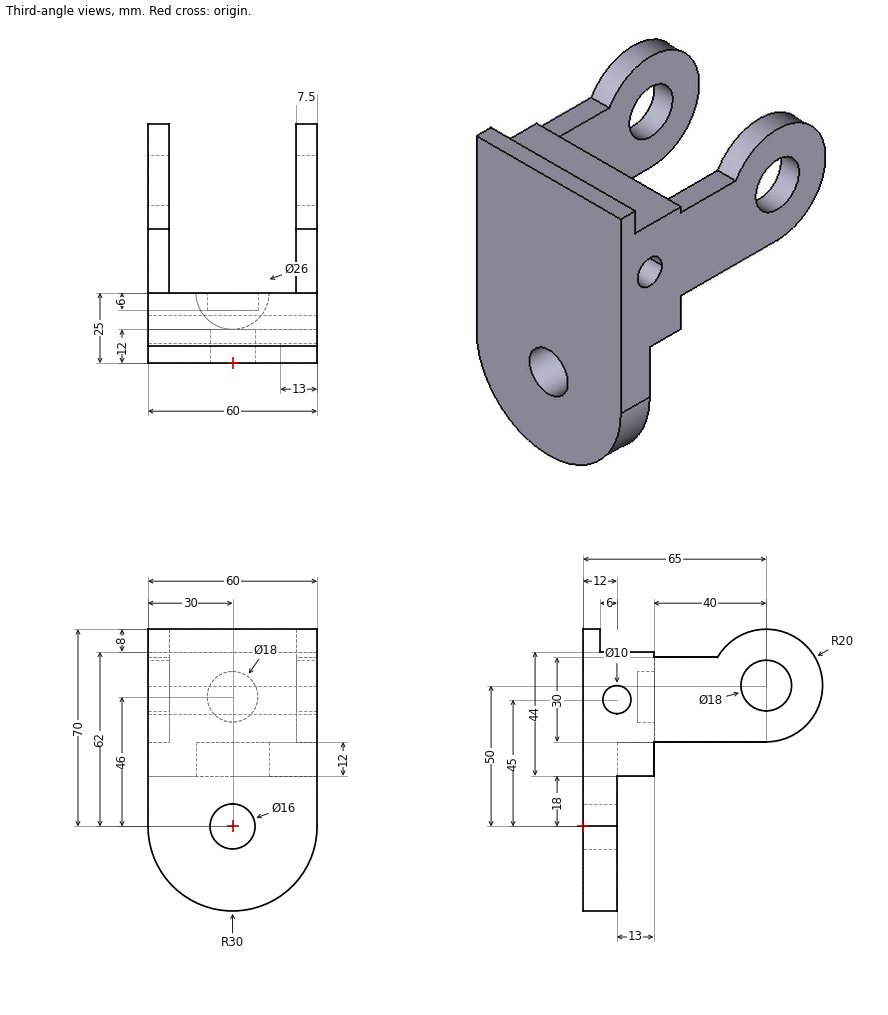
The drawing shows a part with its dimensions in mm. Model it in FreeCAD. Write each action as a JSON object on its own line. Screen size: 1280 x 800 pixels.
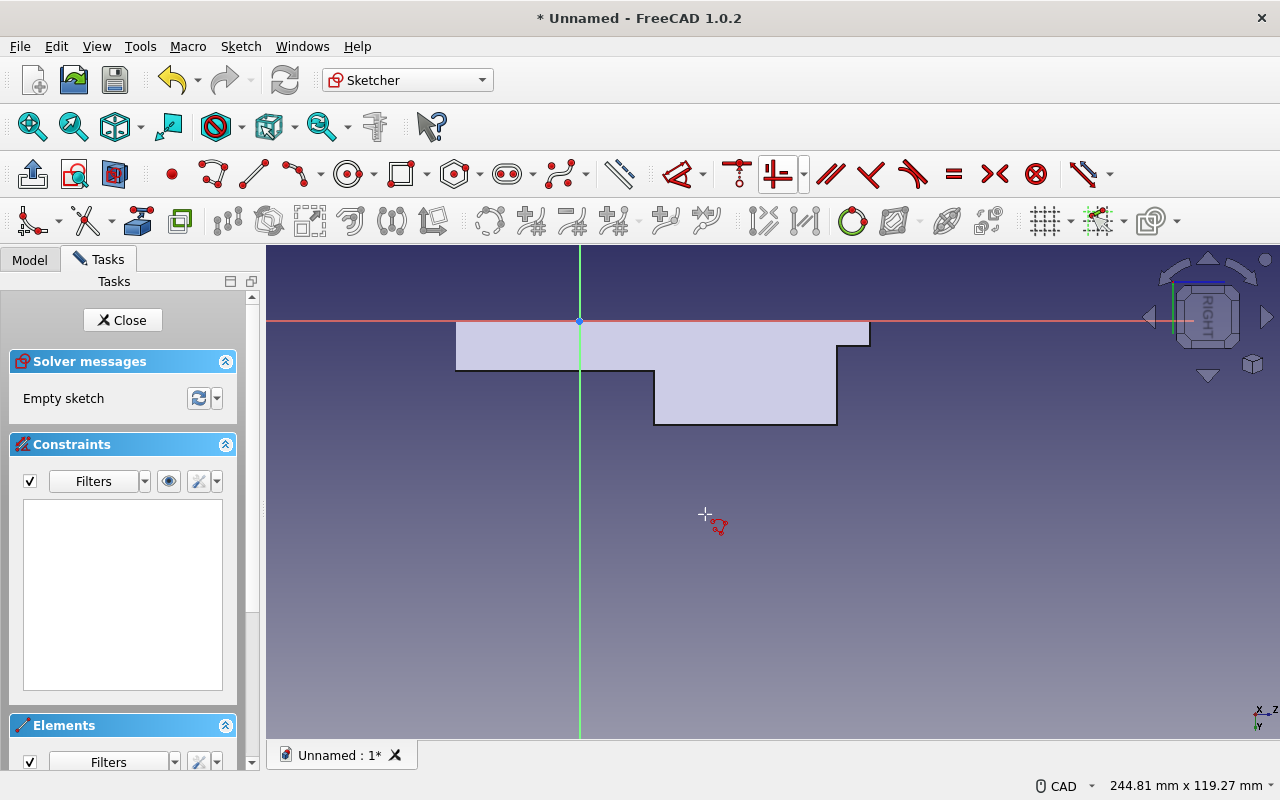
{"action": "left_click", "coordinate": [828, 519]}
{"action": "left_click", "coordinate": [828, 425]}
{"action": "left_click", "coordinate": [704, 425]}
{"action": "left_click", "coordinate": [704, 591]}
{"action": "right_click", "coordinate": [704, 591]}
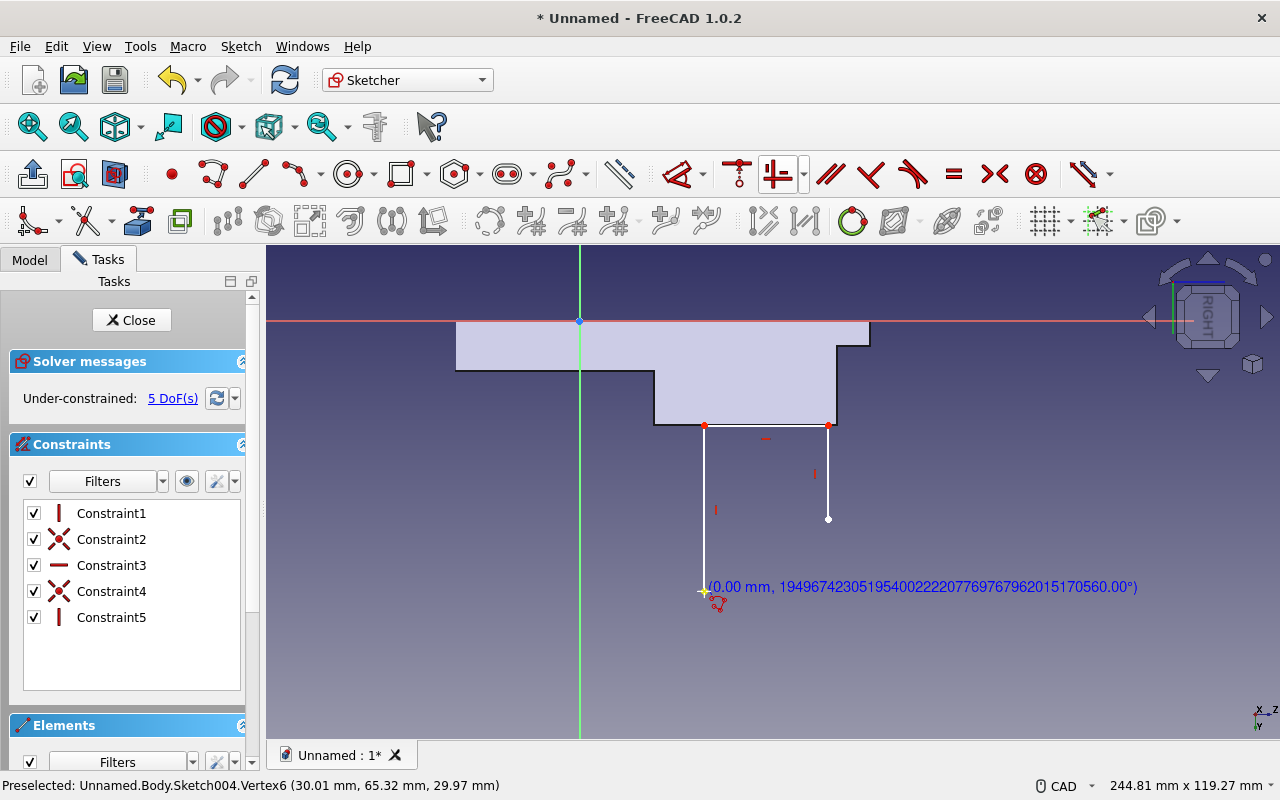
{"action": "left_click", "coordinate": [294, 174]}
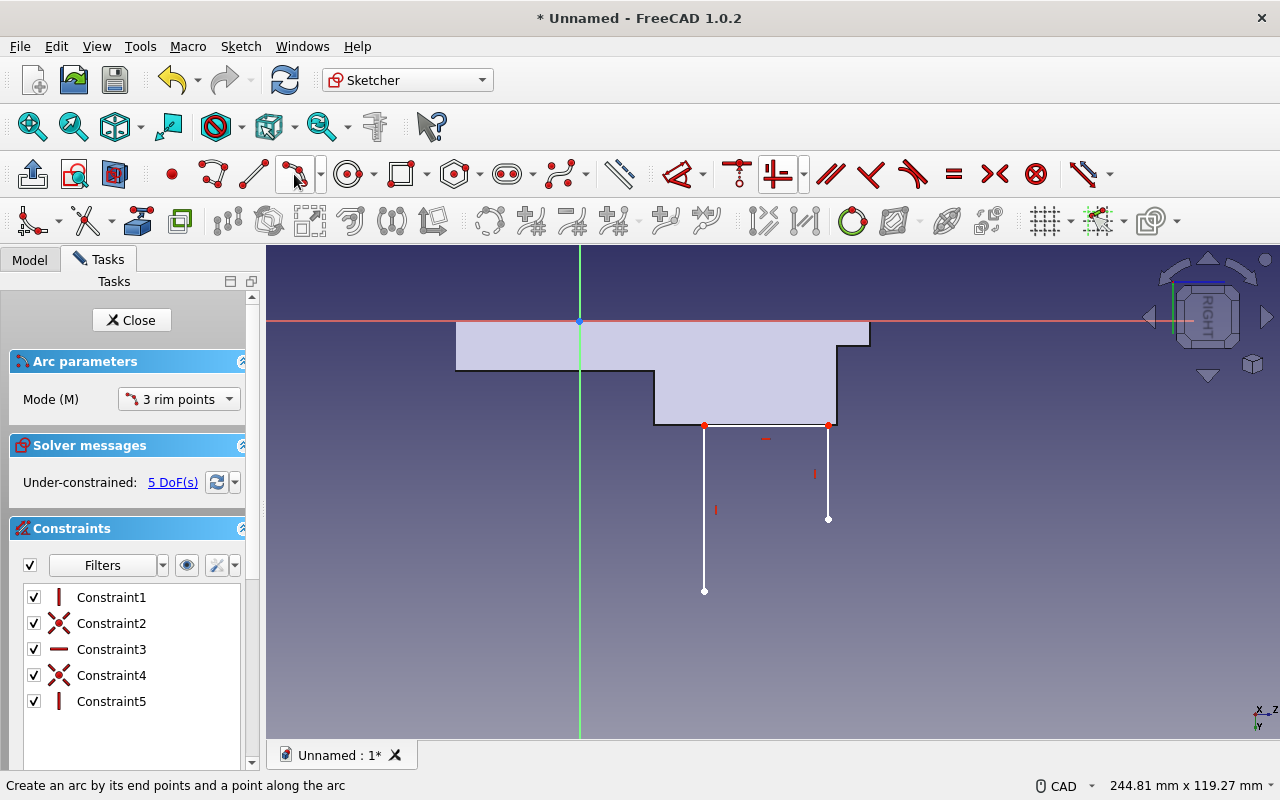
{"action": "left_click", "coordinate": [704, 592]}
{"action": "left_click", "coordinate": [828, 520]}
{"action": "left_click", "coordinate": [828, 662]}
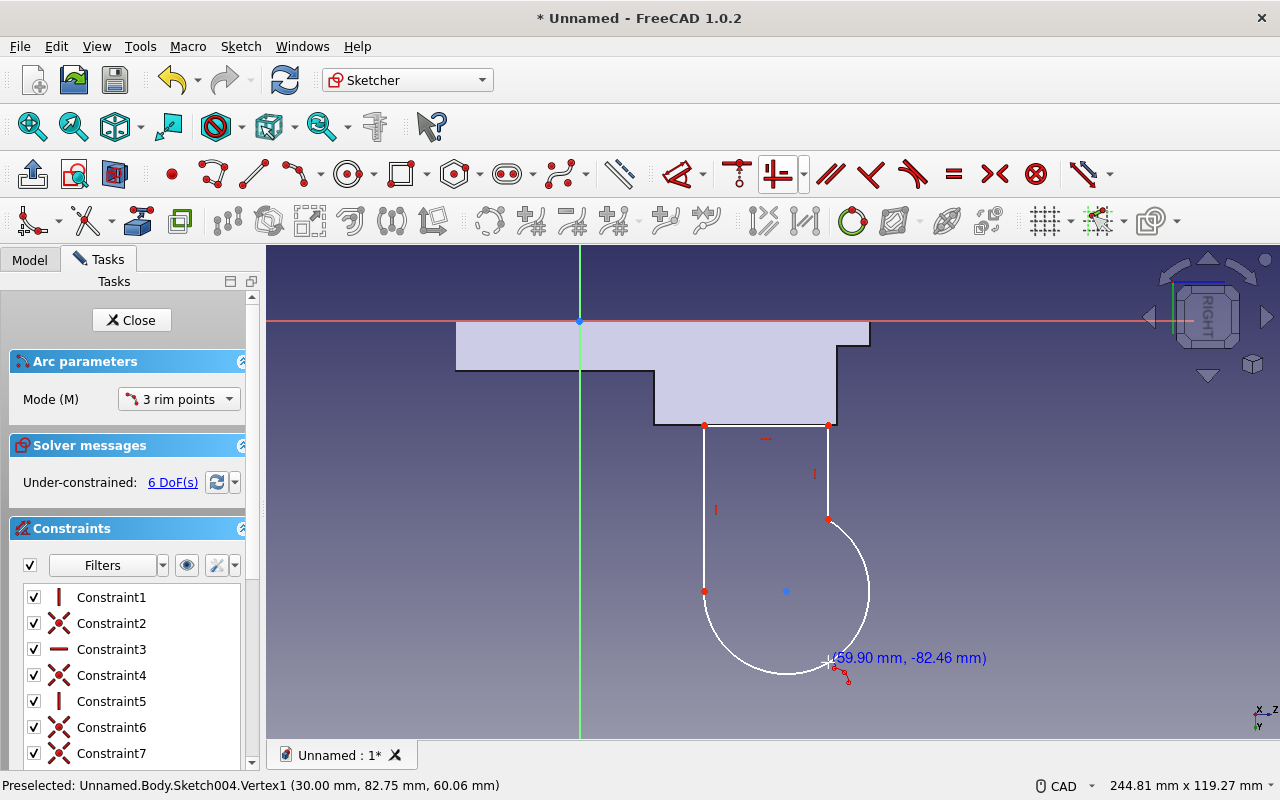
{"action": "left_click", "coordinate": [348, 174]}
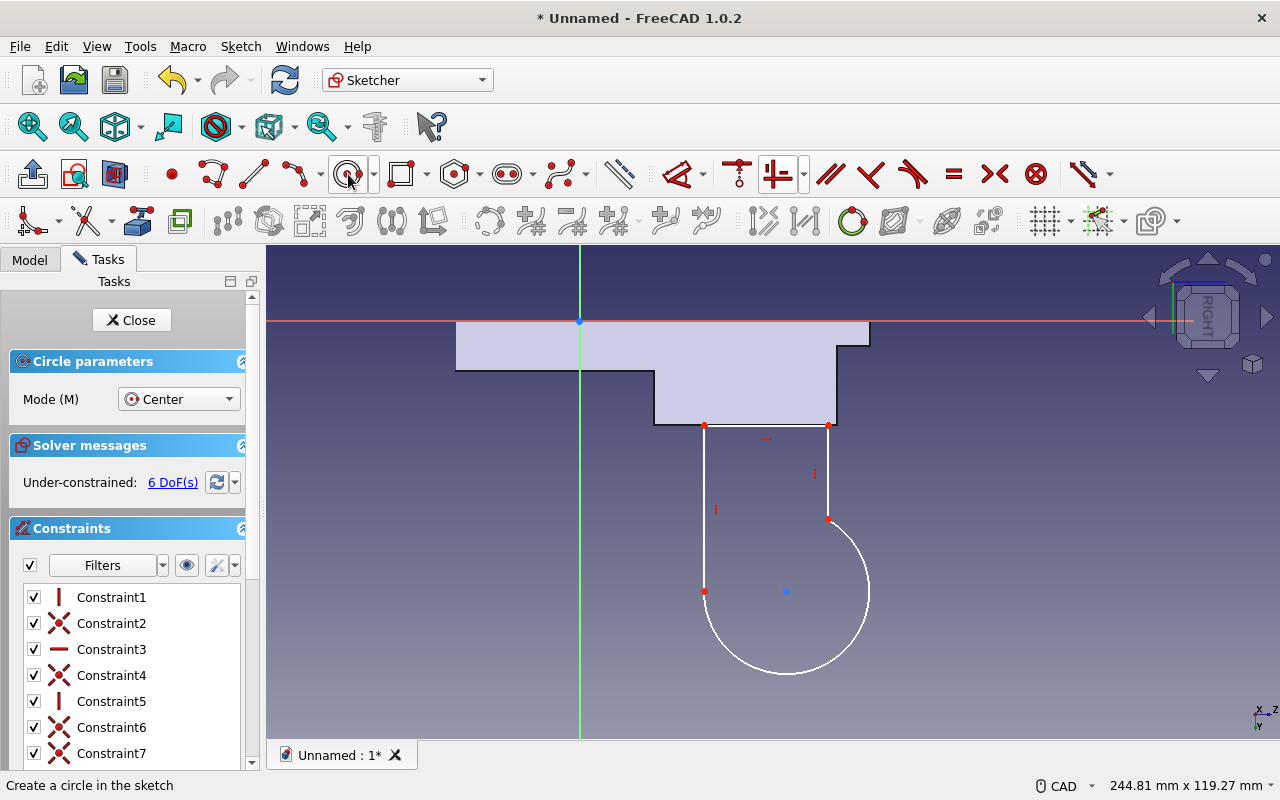
{"action": "left_click", "coordinate": [787, 591]}
{"action": "left_click", "coordinate": [813, 564]}
{"action": "key", "text": "Escape"}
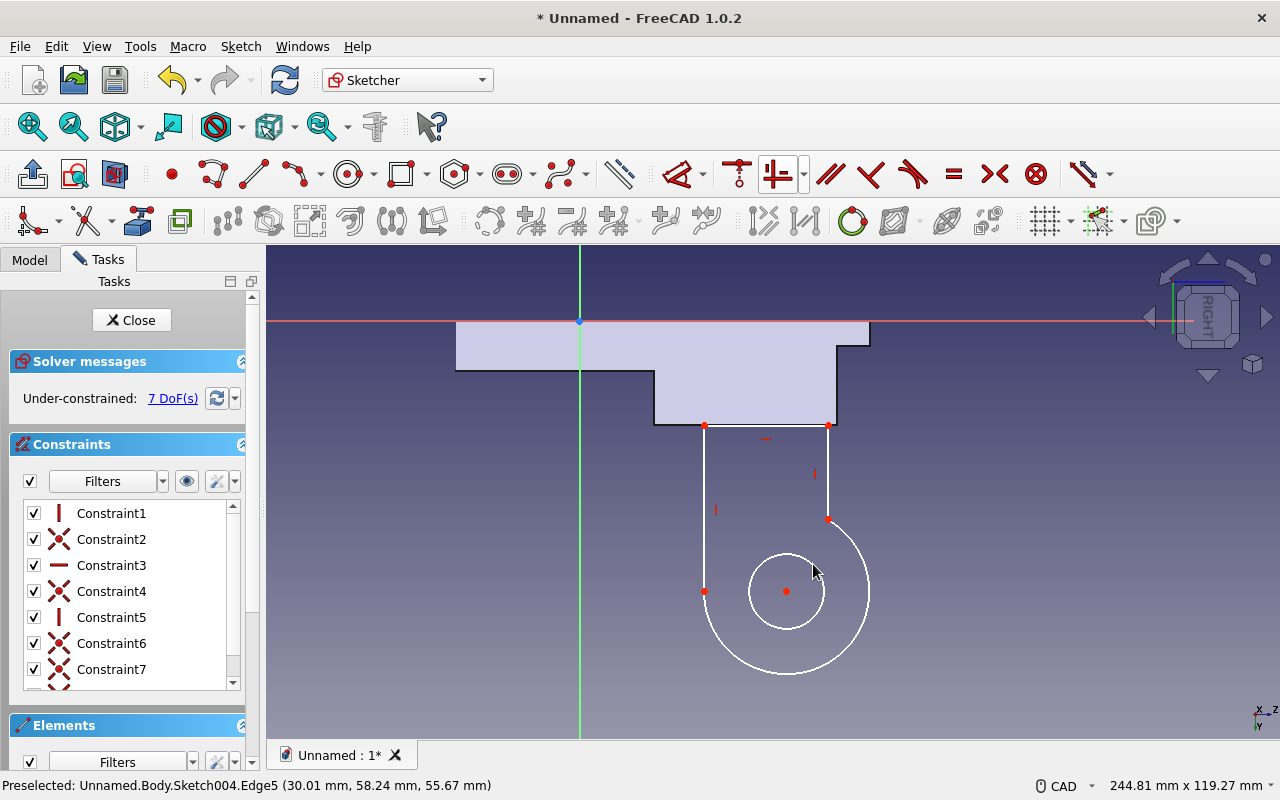
{"action": "left_click", "coordinate": [704, 476]}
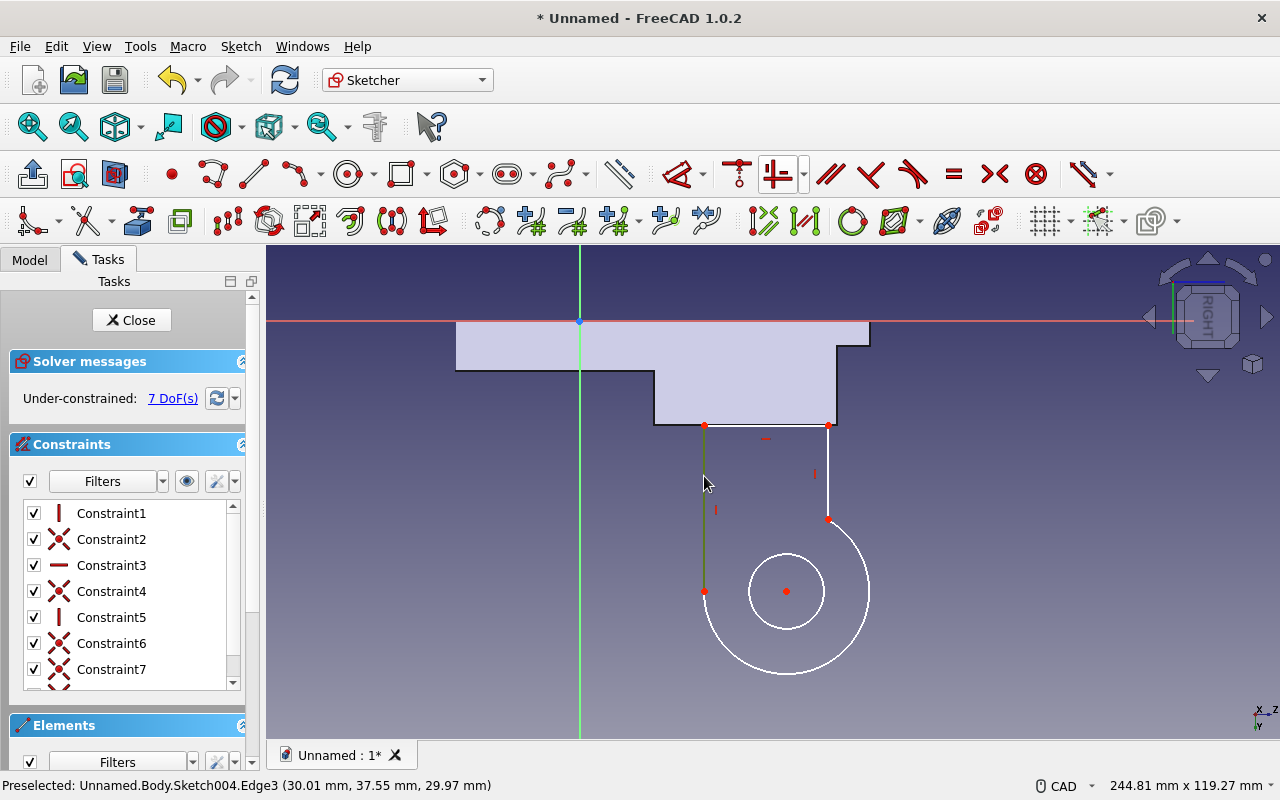
{"action": "left_click", "coordinate": [761, 670]}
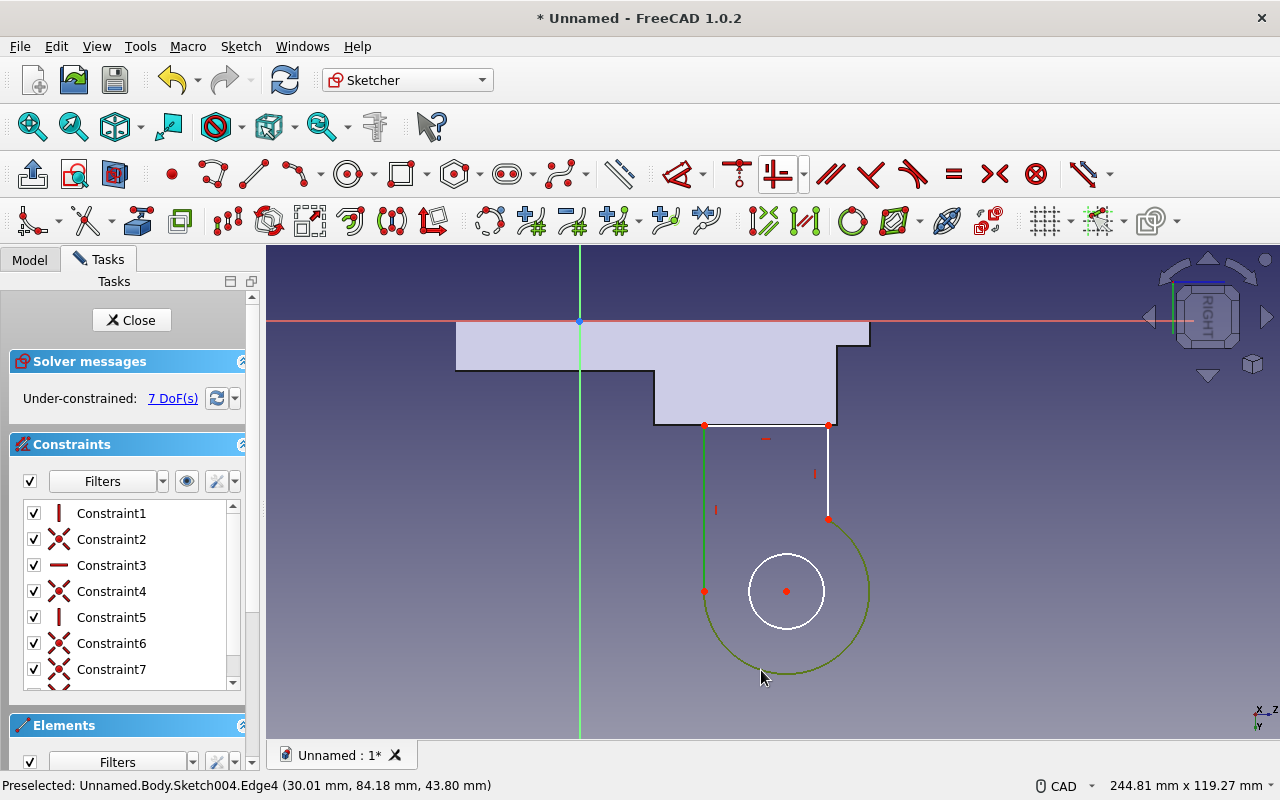
{"action": "key", "text": "t"}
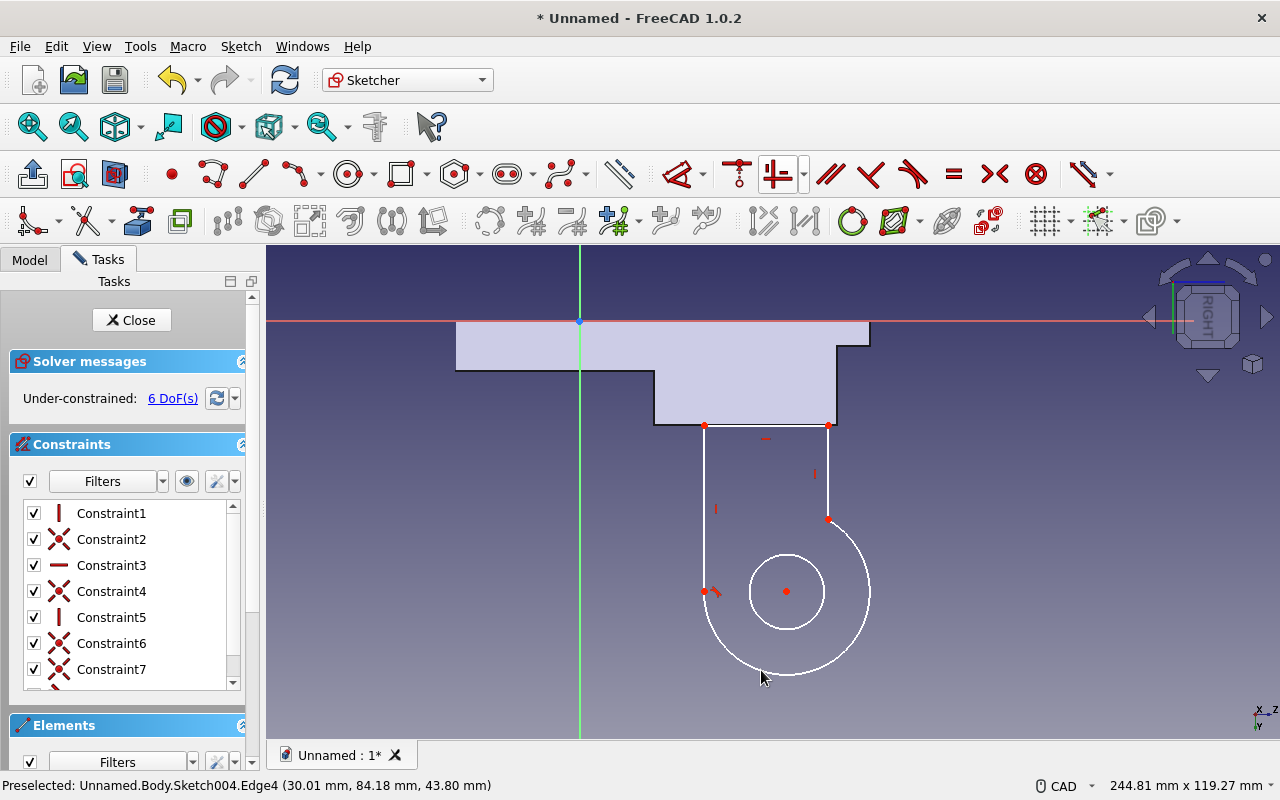
{"action": "key", "text": "d"}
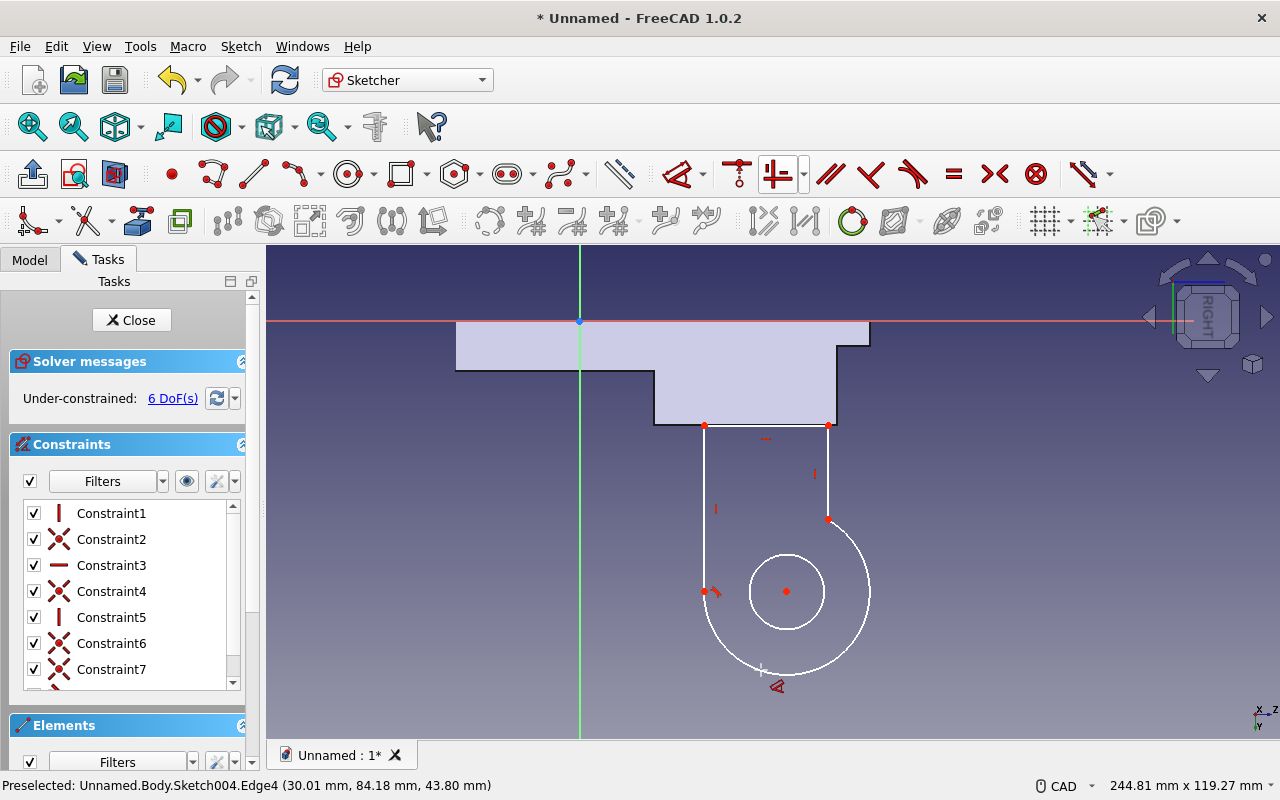
{"action": "left_click", "coordinate": [761, 671]}
{"action": "left_click", "coordinate": [751, 701]}